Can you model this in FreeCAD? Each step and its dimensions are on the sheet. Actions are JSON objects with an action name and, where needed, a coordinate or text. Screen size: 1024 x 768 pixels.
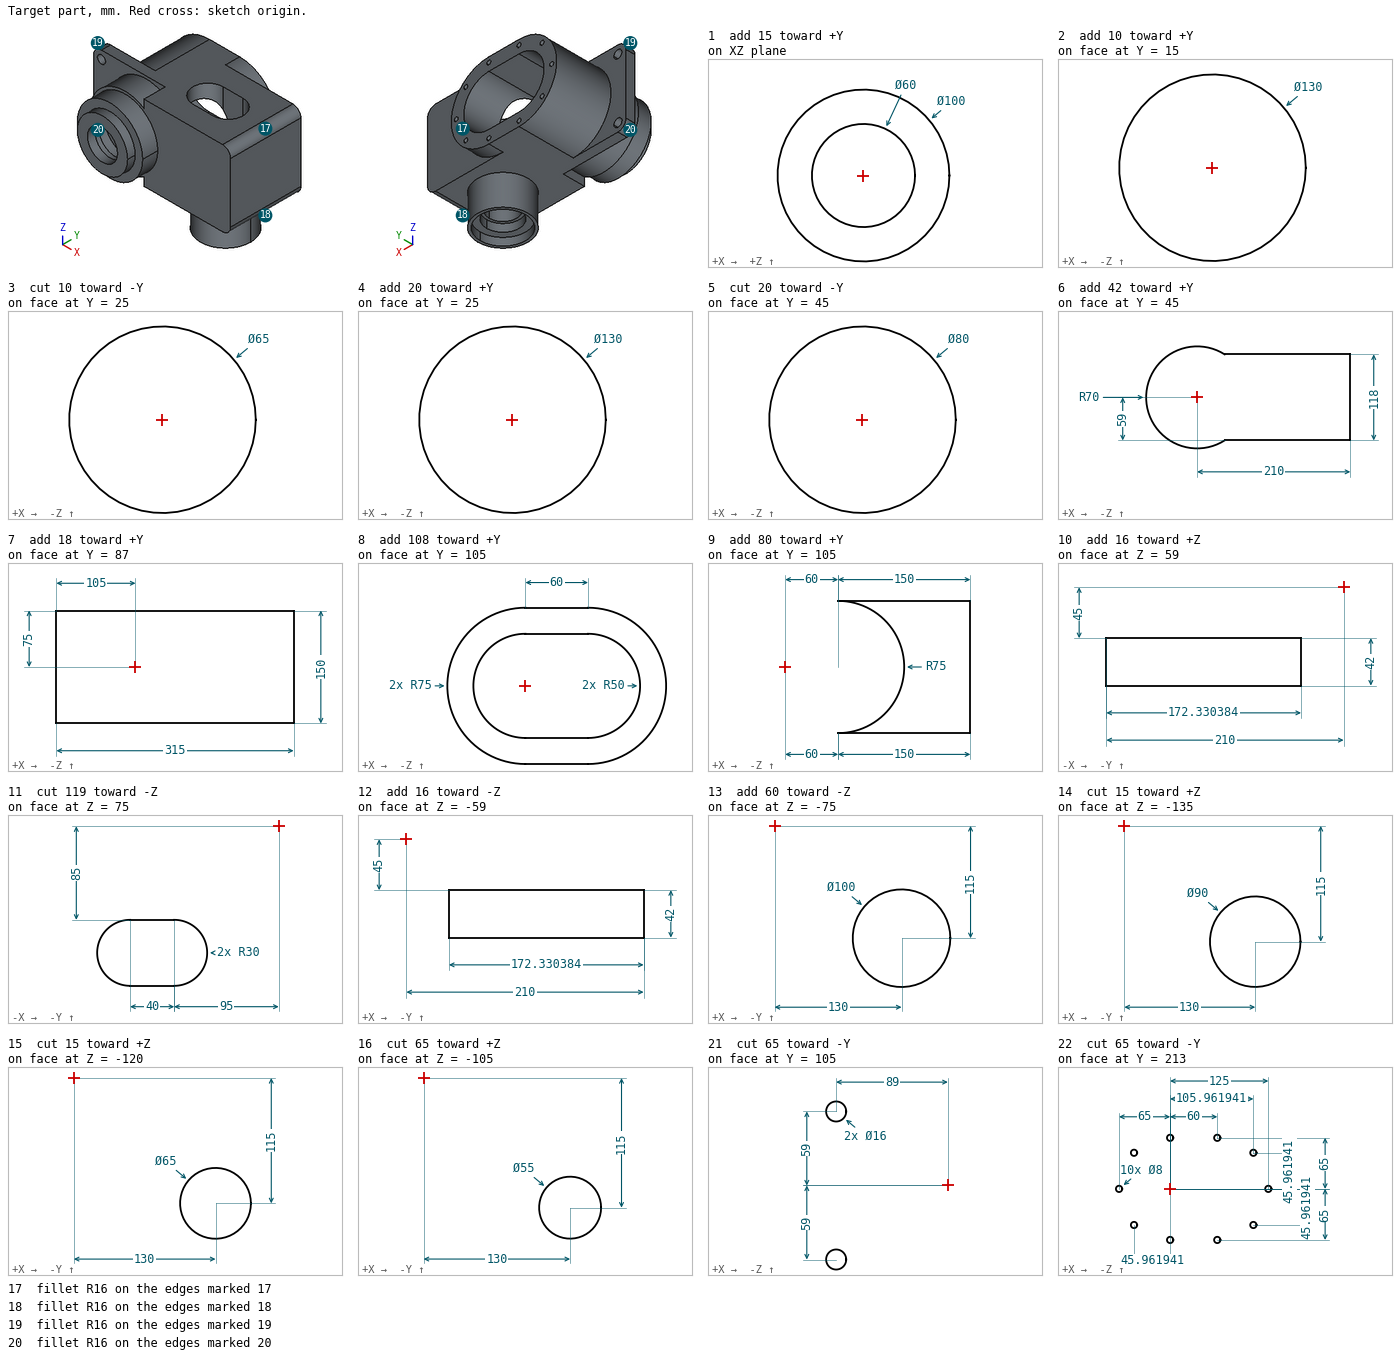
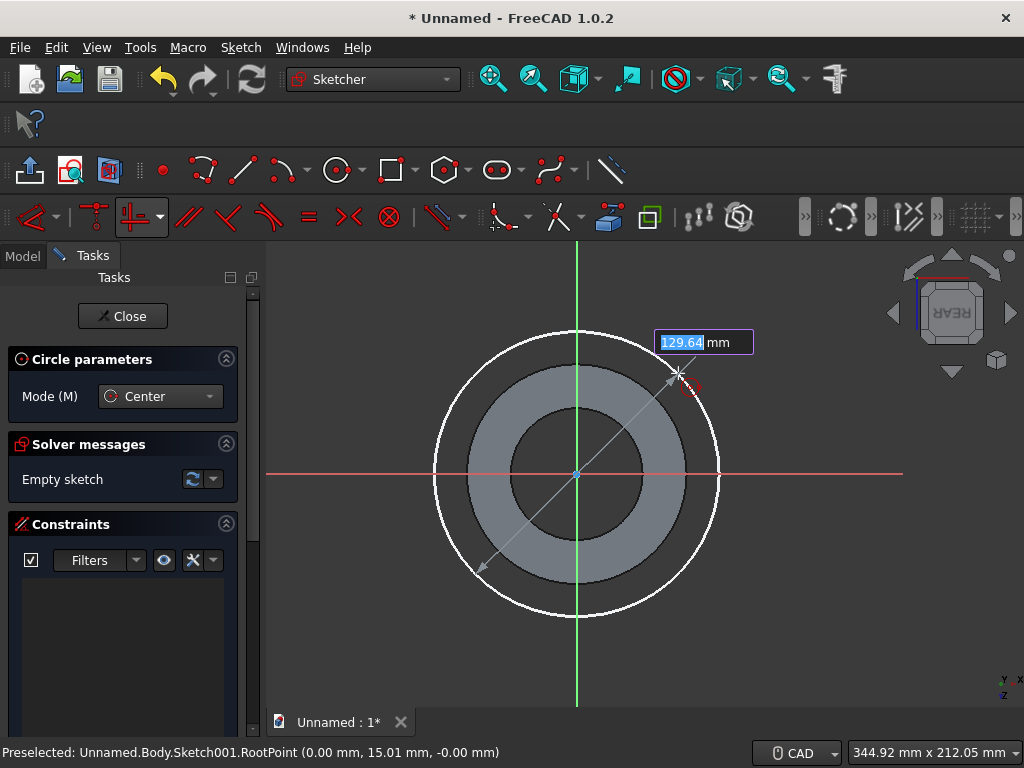
{"action": "type", "text": "130"}
{"action": "key", "text": "Return"}
{"action": "key", "text": "Escape"}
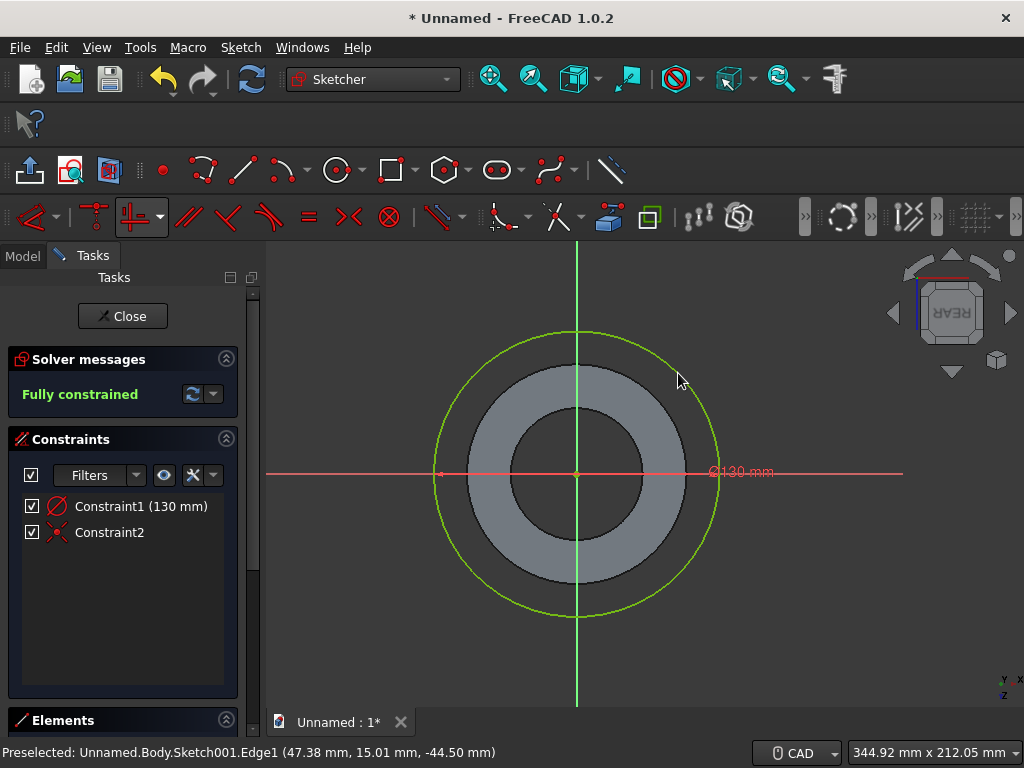
{"action": "left_click", "coordinate": [123, 316]}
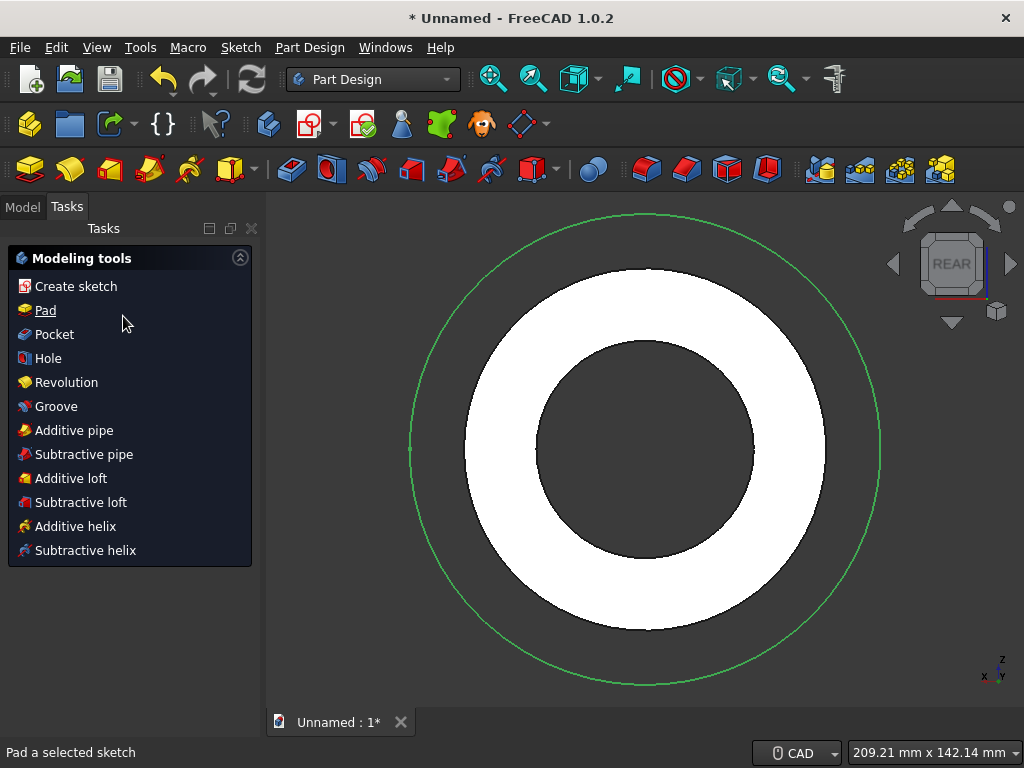
{"action": "left_click", "coordinate": [30, 170]}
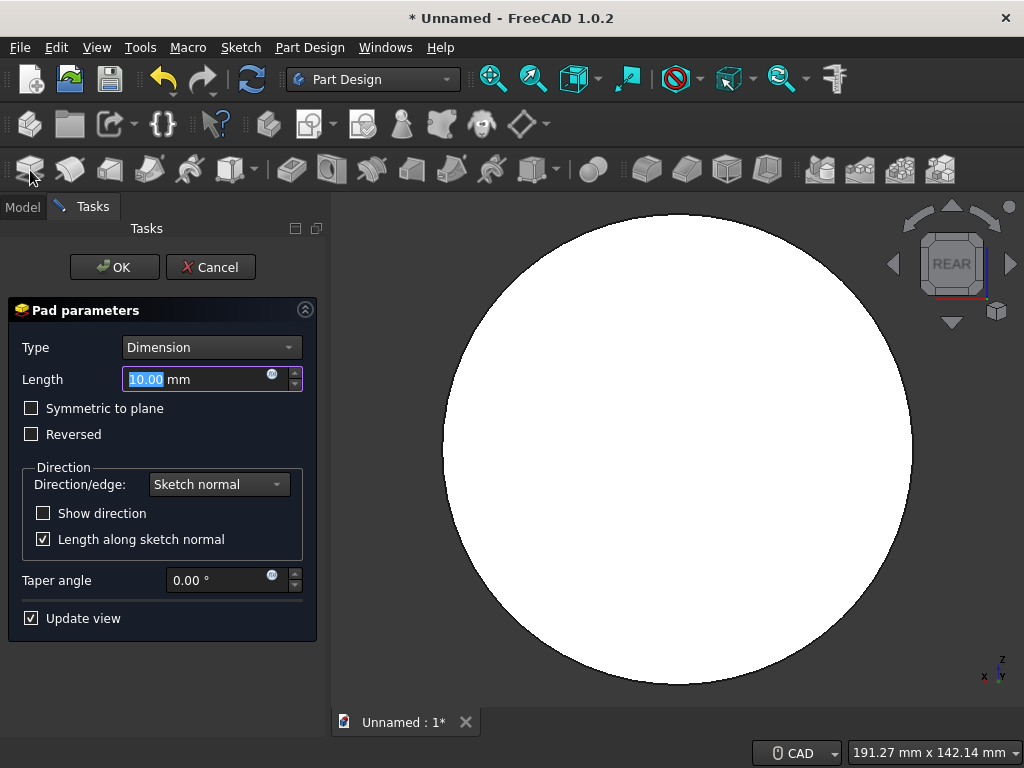
{"action": "type", "text": "10"}
{"action": "key", "text": "Tab"}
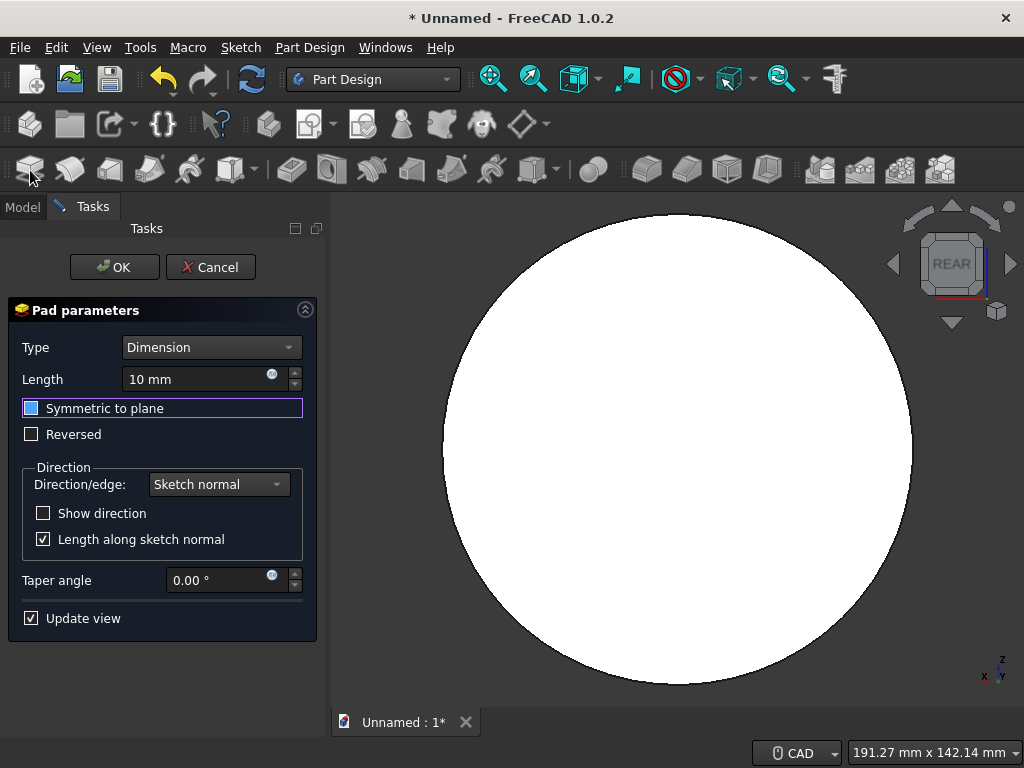
{"action": "left_click", "coordinate": [115, 267]}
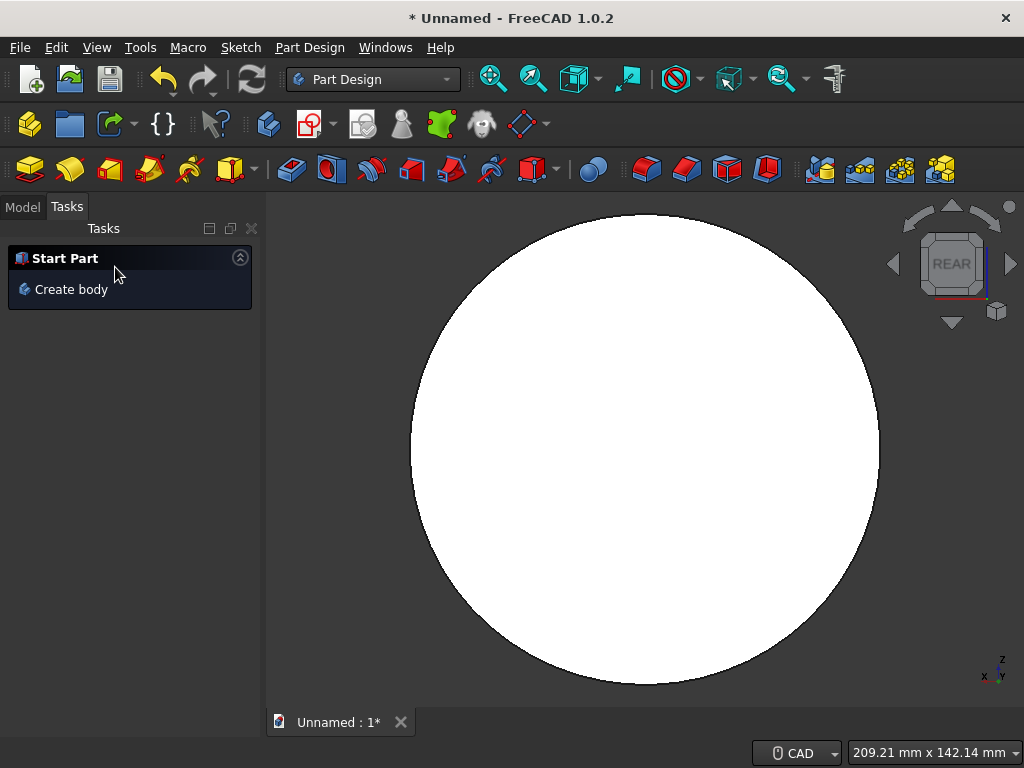
{"action": "left_click", "coordinate": [645, 448]}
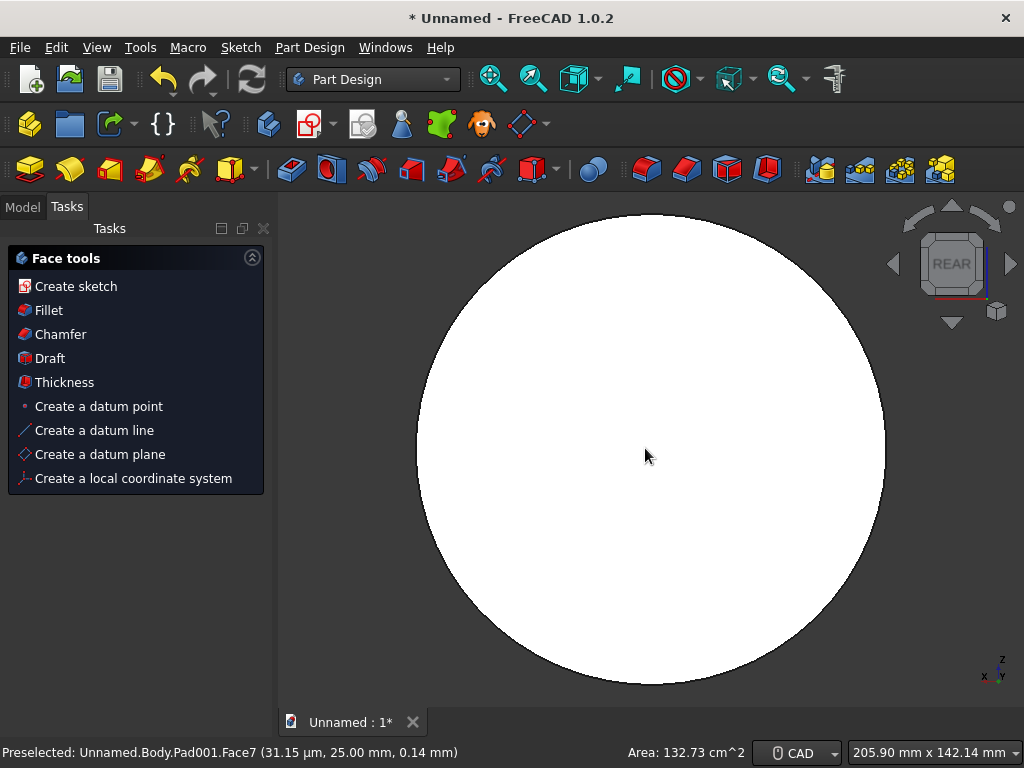
{"action": "left_click", "coordinate": [310, 124]}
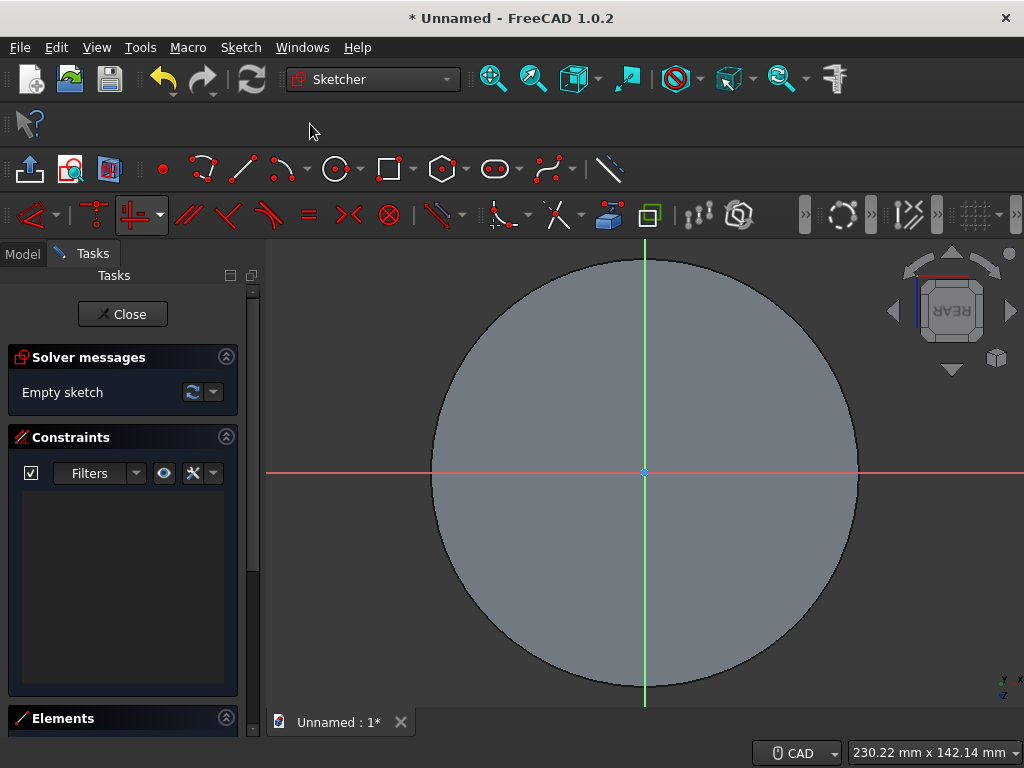
{"action": "scroll", "coordinate": [784, 473], "scroll_direction": "up", "scroll_amount": 2}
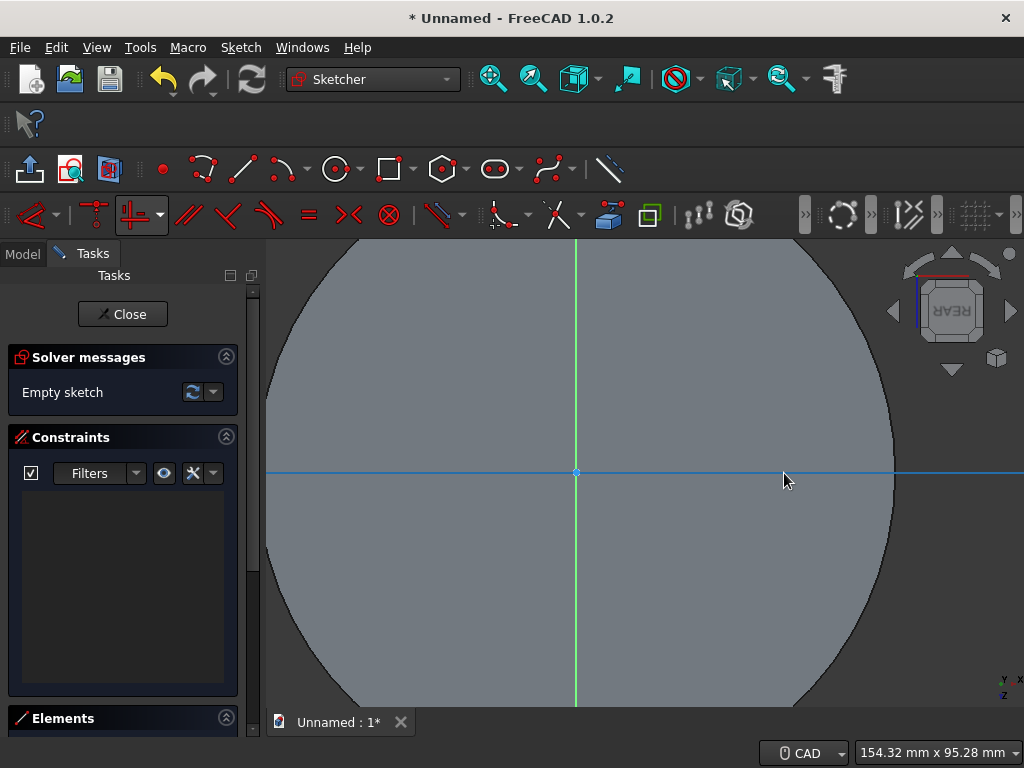
{"action": "left_click", "coordinate": [336, 170]}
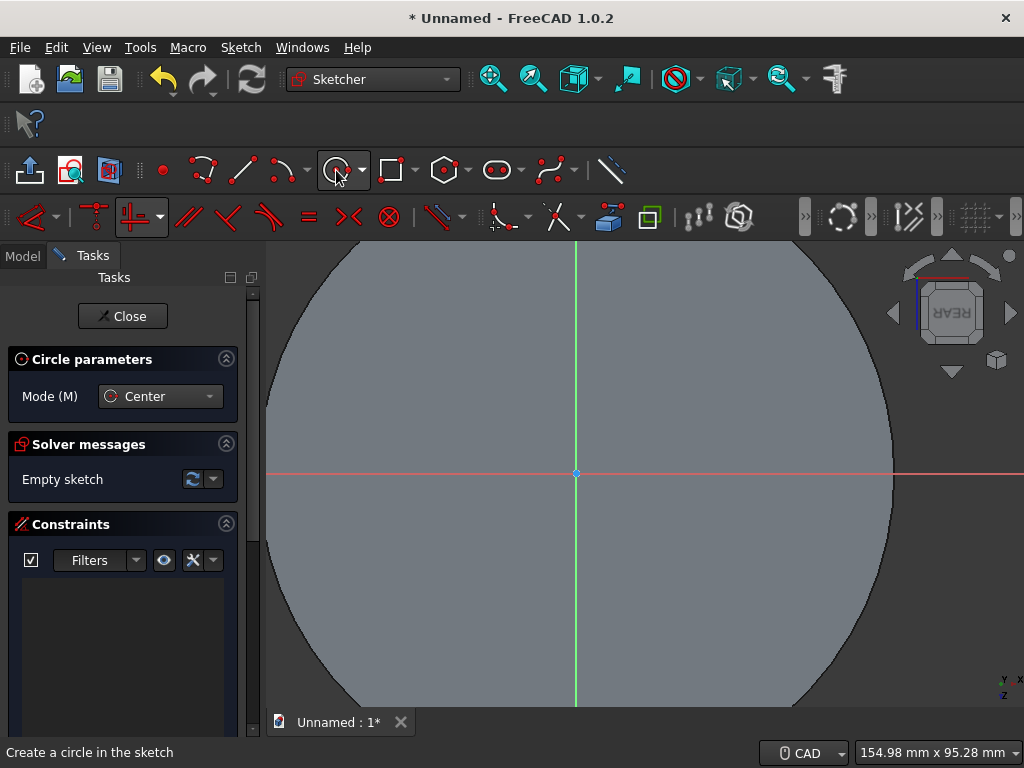
{"action": "left_click", "coordinate": [576, 474]}
{"action": "mouse_move", "coordinate": [689, 361]}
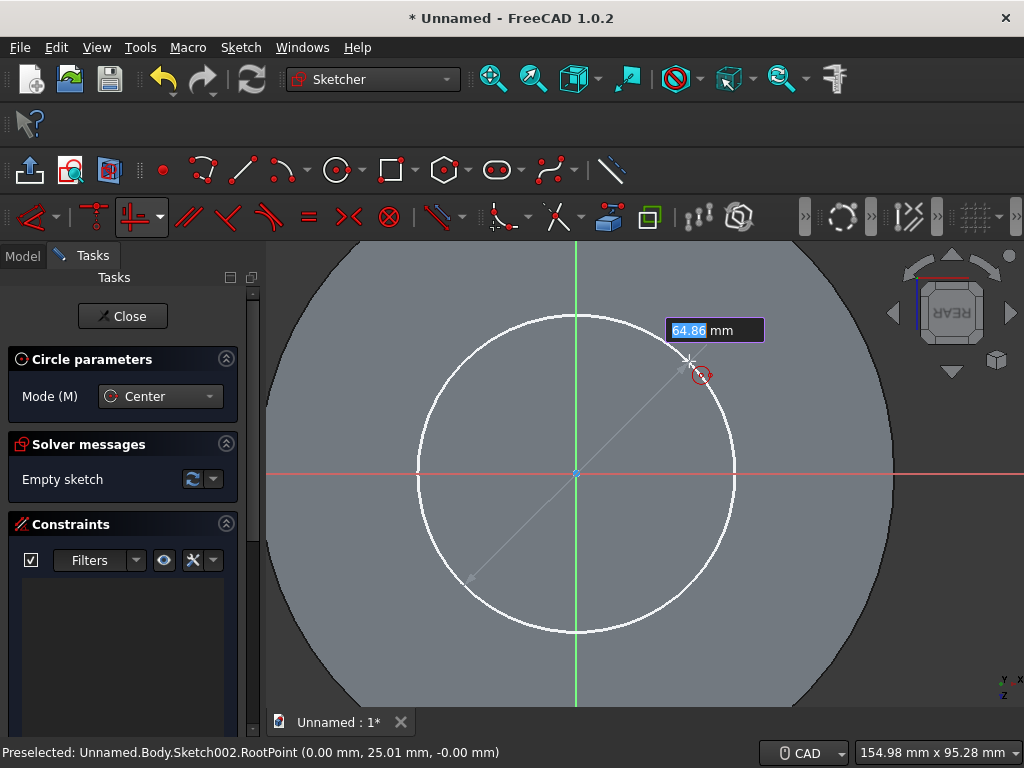
{"action": "type", "text": "65"}
{"action": "key", "text": "Return"}
{"action": "key", "text": "Escape"}